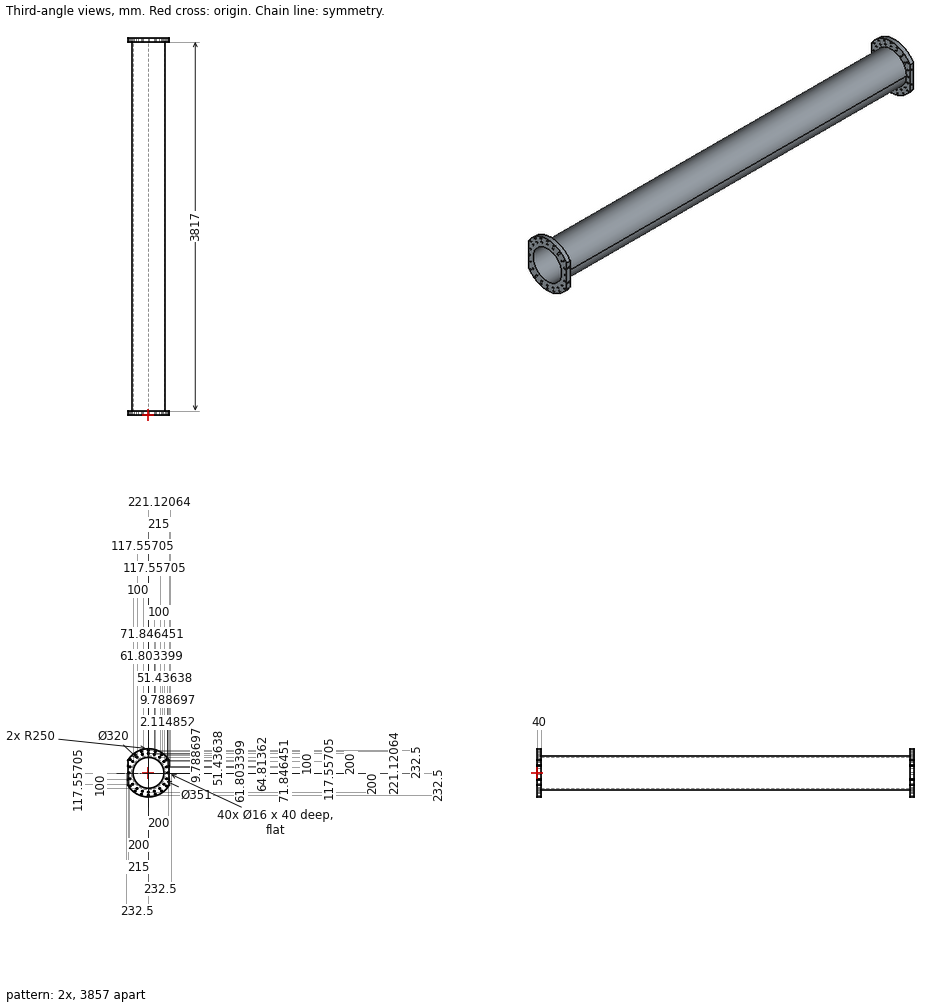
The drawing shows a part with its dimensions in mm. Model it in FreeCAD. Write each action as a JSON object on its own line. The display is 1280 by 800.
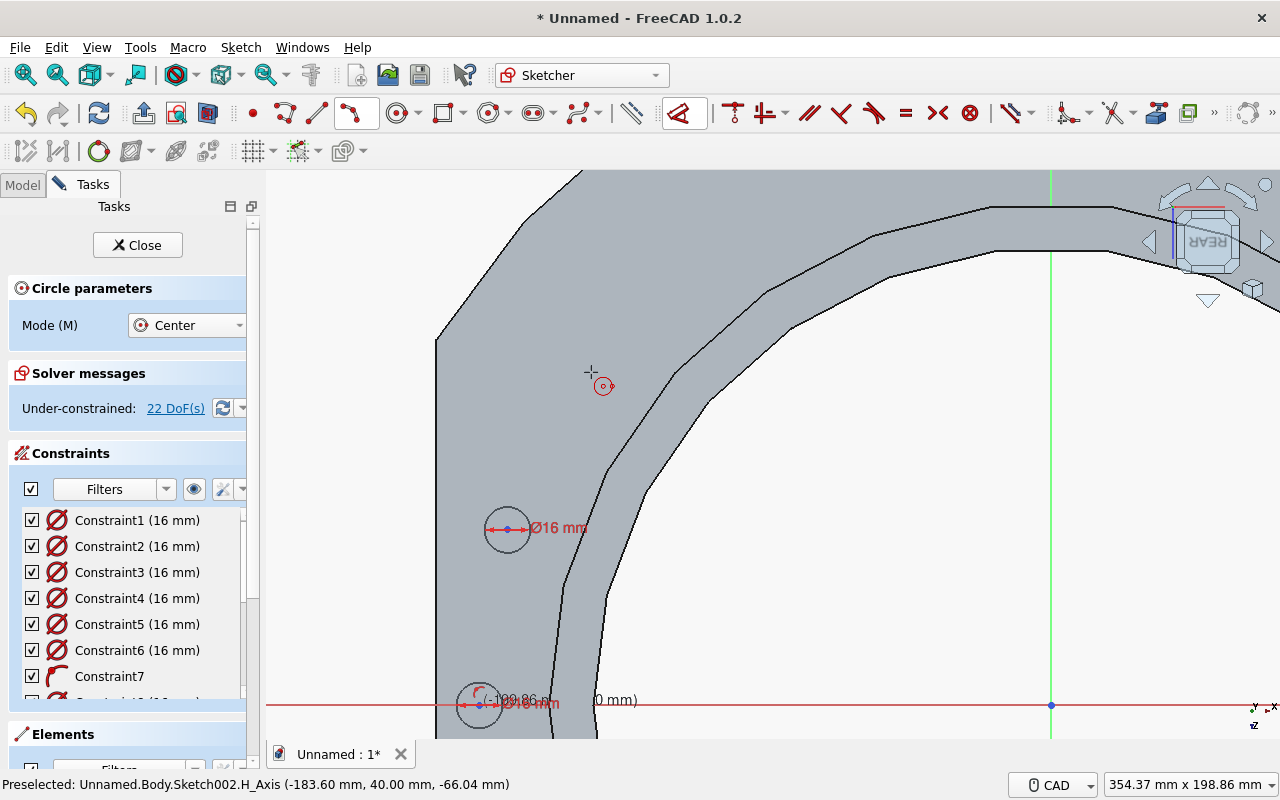
{"action": "left_click", "coordinate": [588, 369]}
{"action": "mouse_move", "coordinate": [605, 353]}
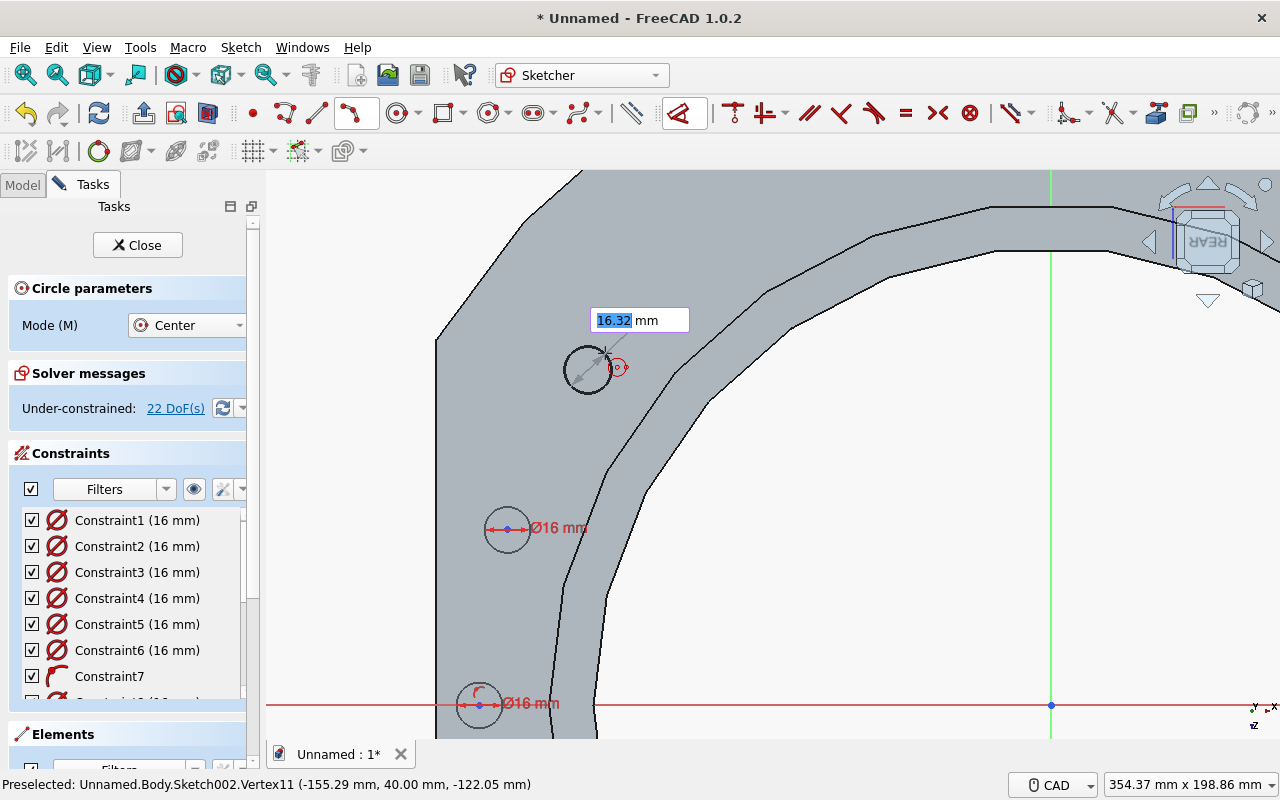
{"action": "type", "text": "16"}
{"action": "key", "text": "Return"}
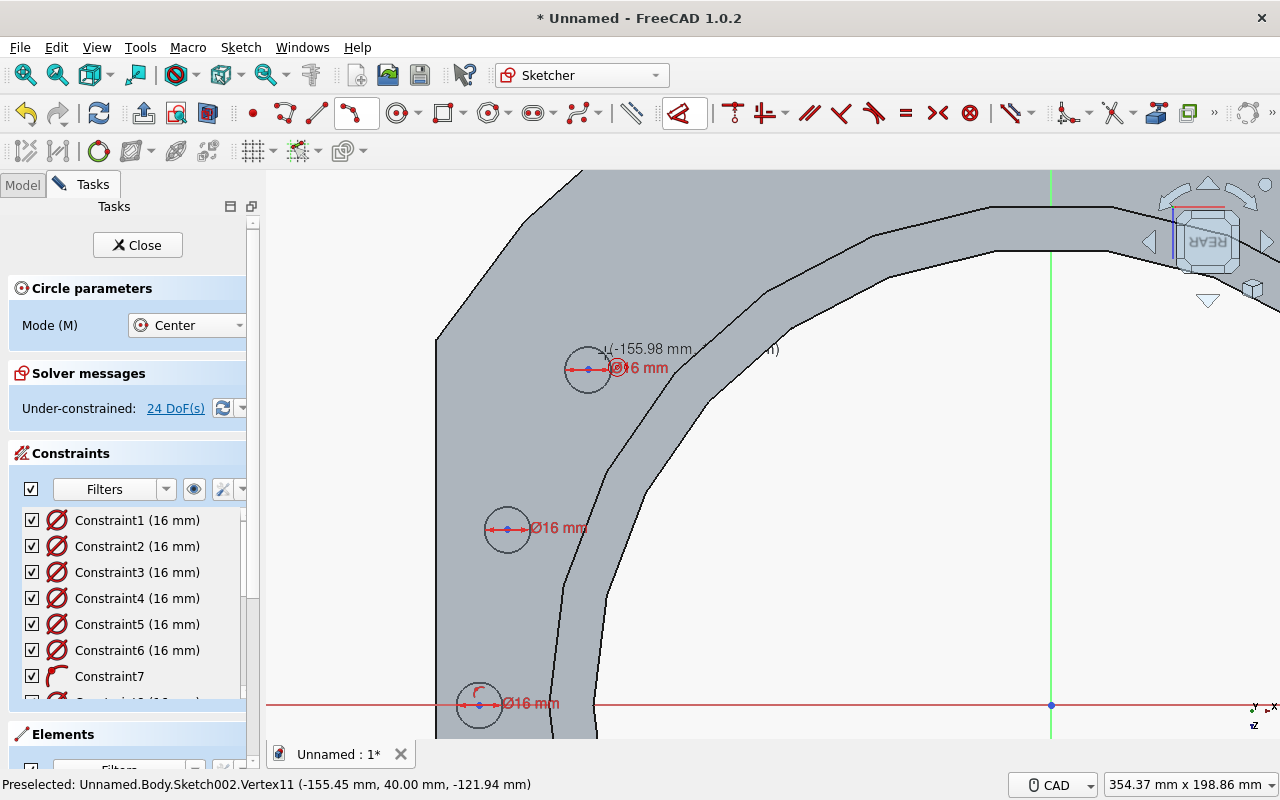
{"action": "left_click", "coordinate": [715, 242]}
{"action": "mouse_move", "coordinate": [731, 226]}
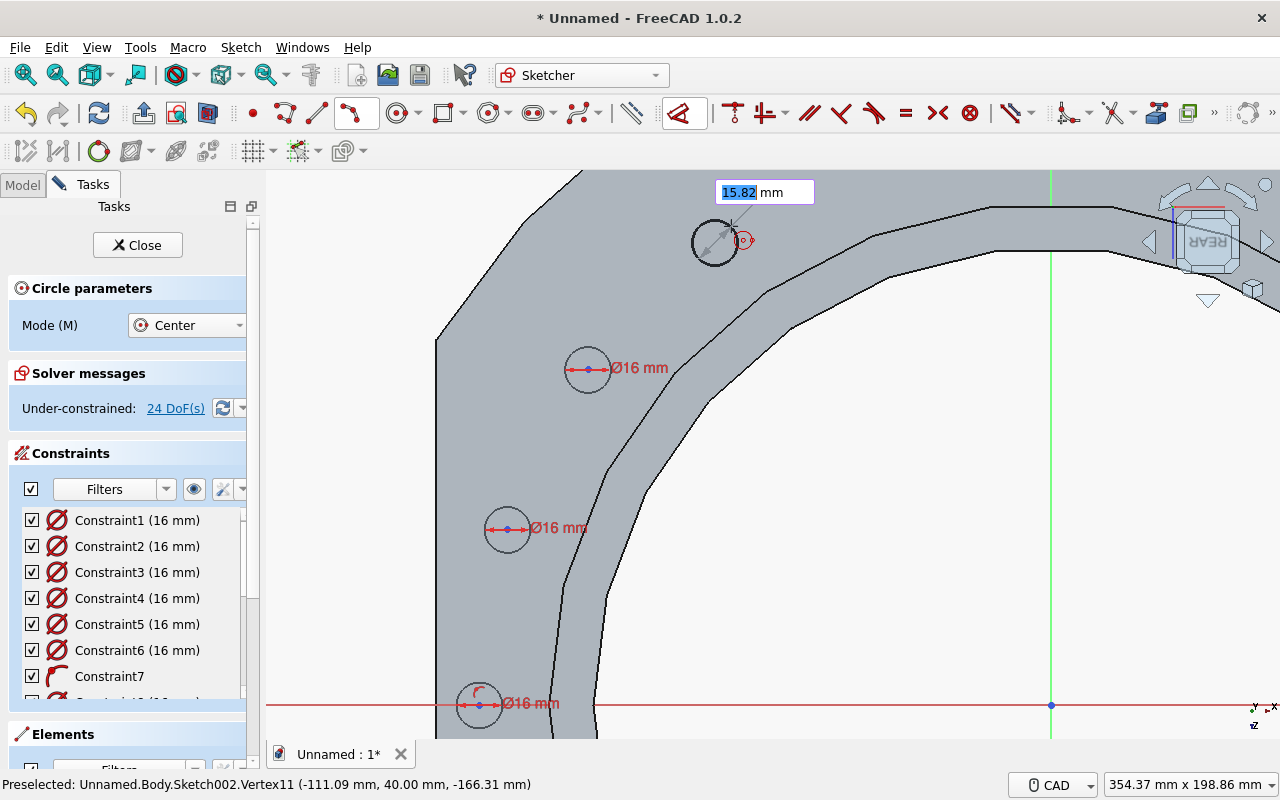
{"action": "type", "text": "16"}
{"action": "key", "text": "Return"}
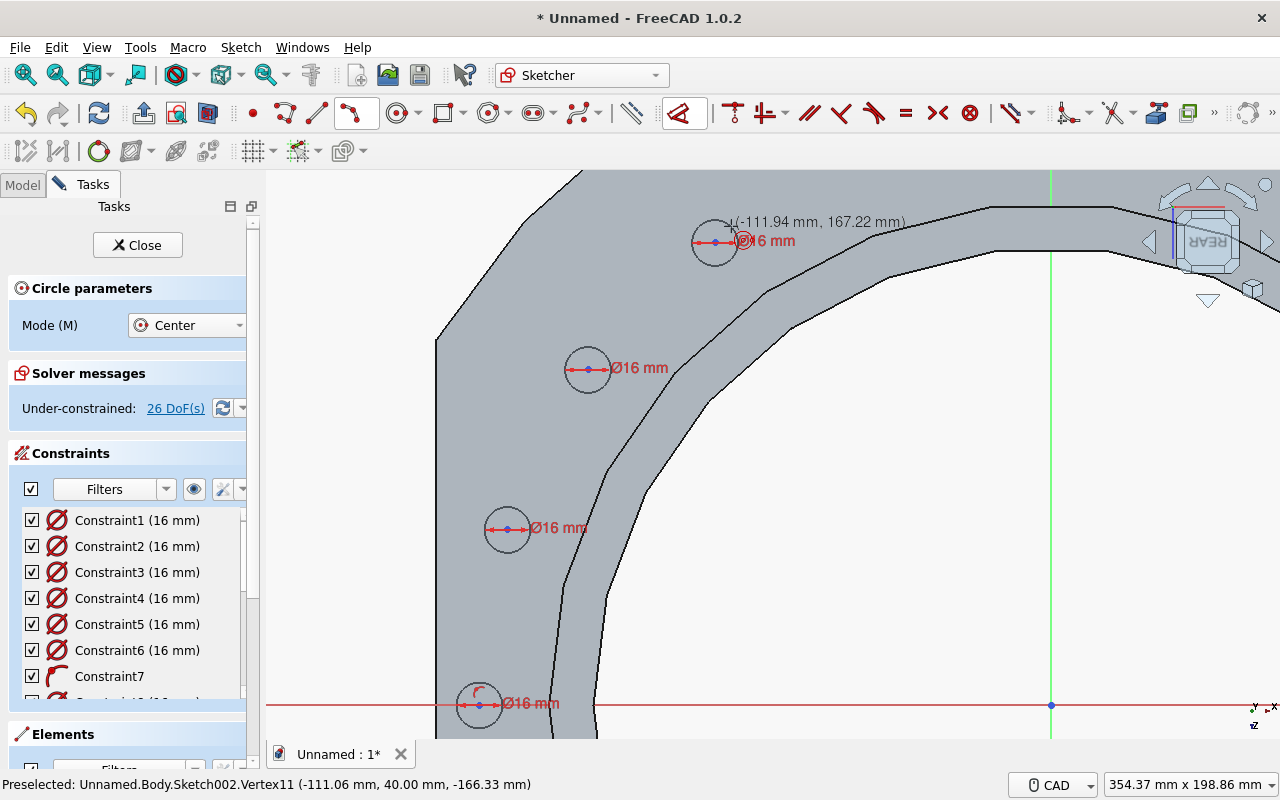
{"action": "scroll", "coordinate": [591, 372], "scroll_direction": "down", "scroll_amount": 7}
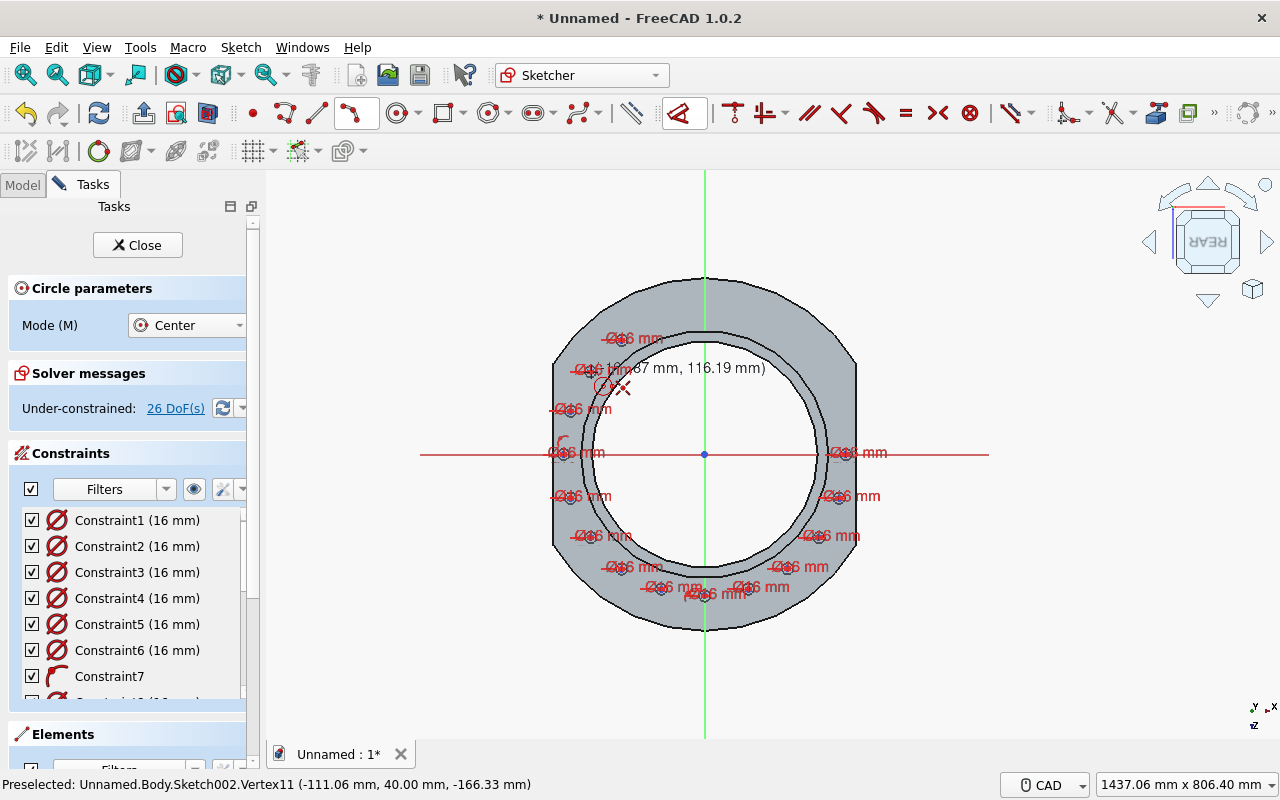
{"action": "scroll", "coordinate": [661, 320], "scroll_direction": "up", "scroll_amount": 7}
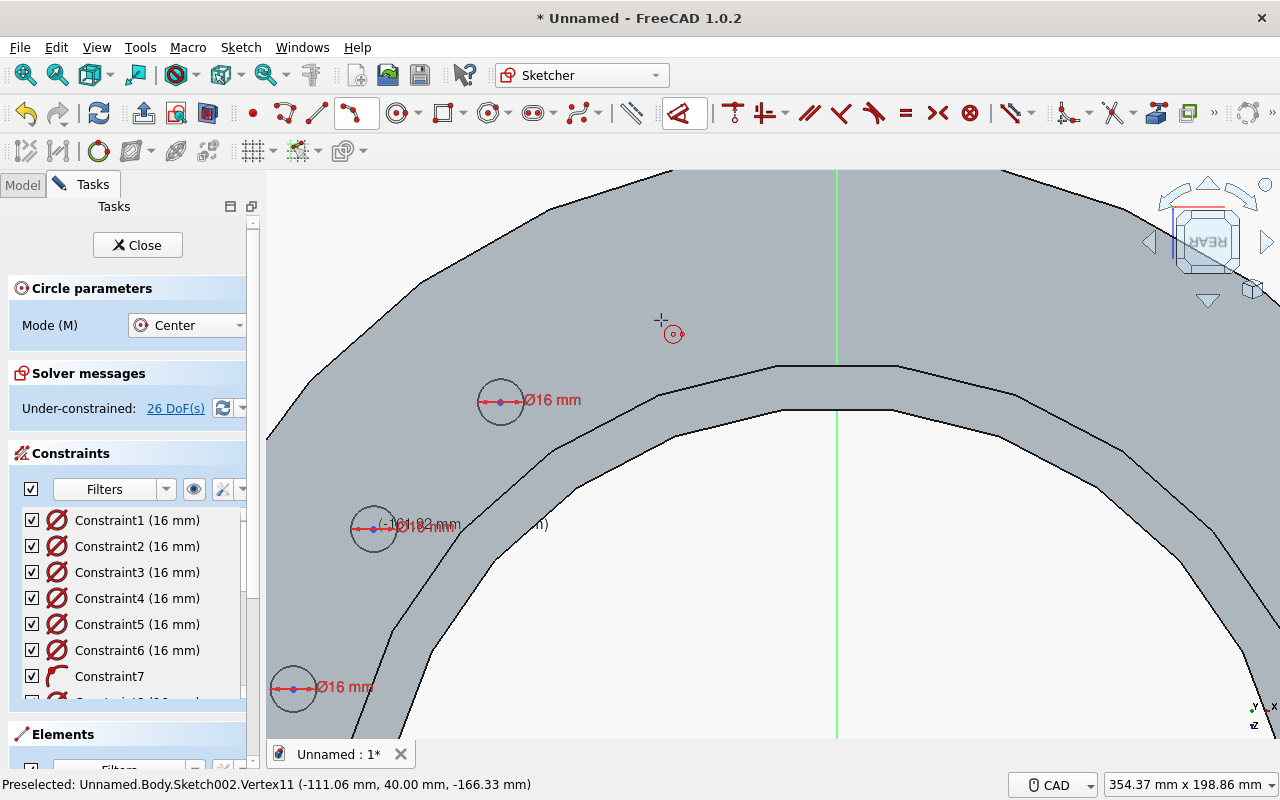
{"action": "left_click", "coordinate": [660, 320]}
{"action": "mouse_move", "coordinate": [677, 304]}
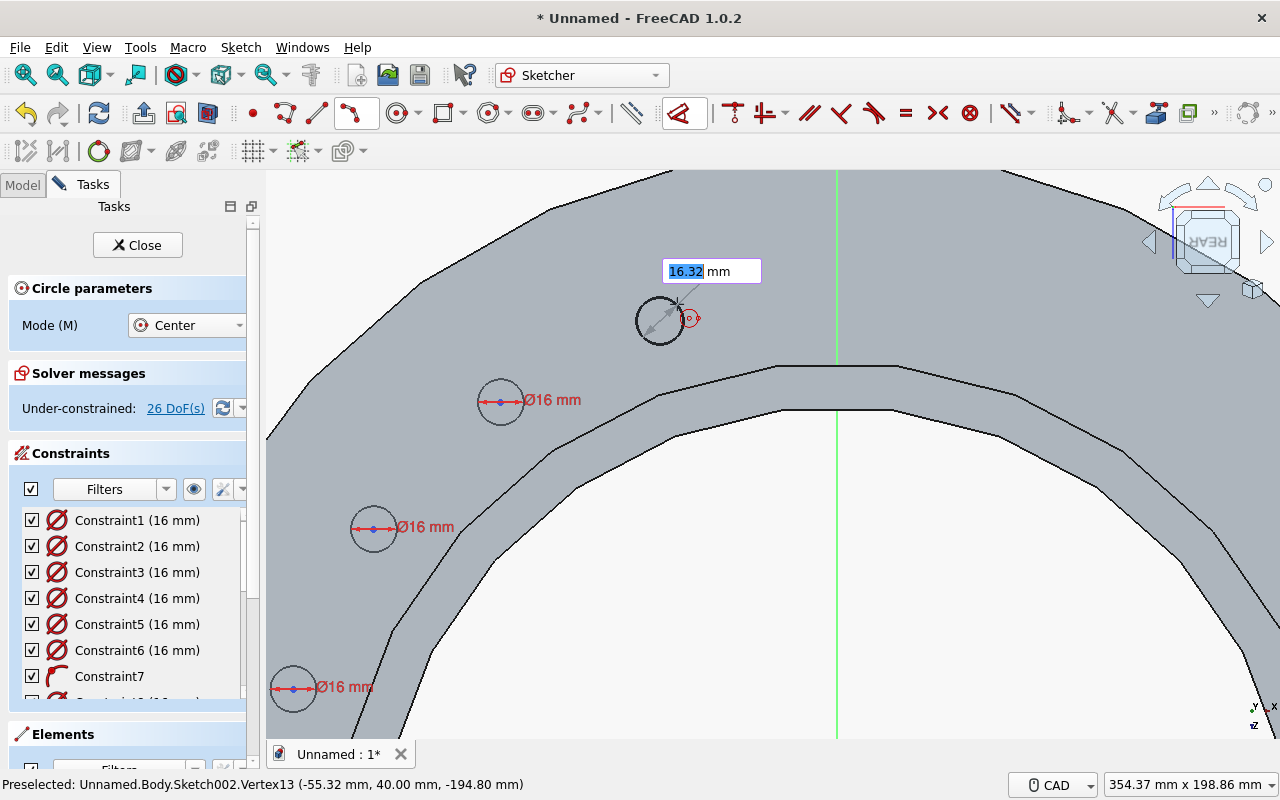
{"action": "type", "text": "16"}
{"action": "key", "text": "Return"}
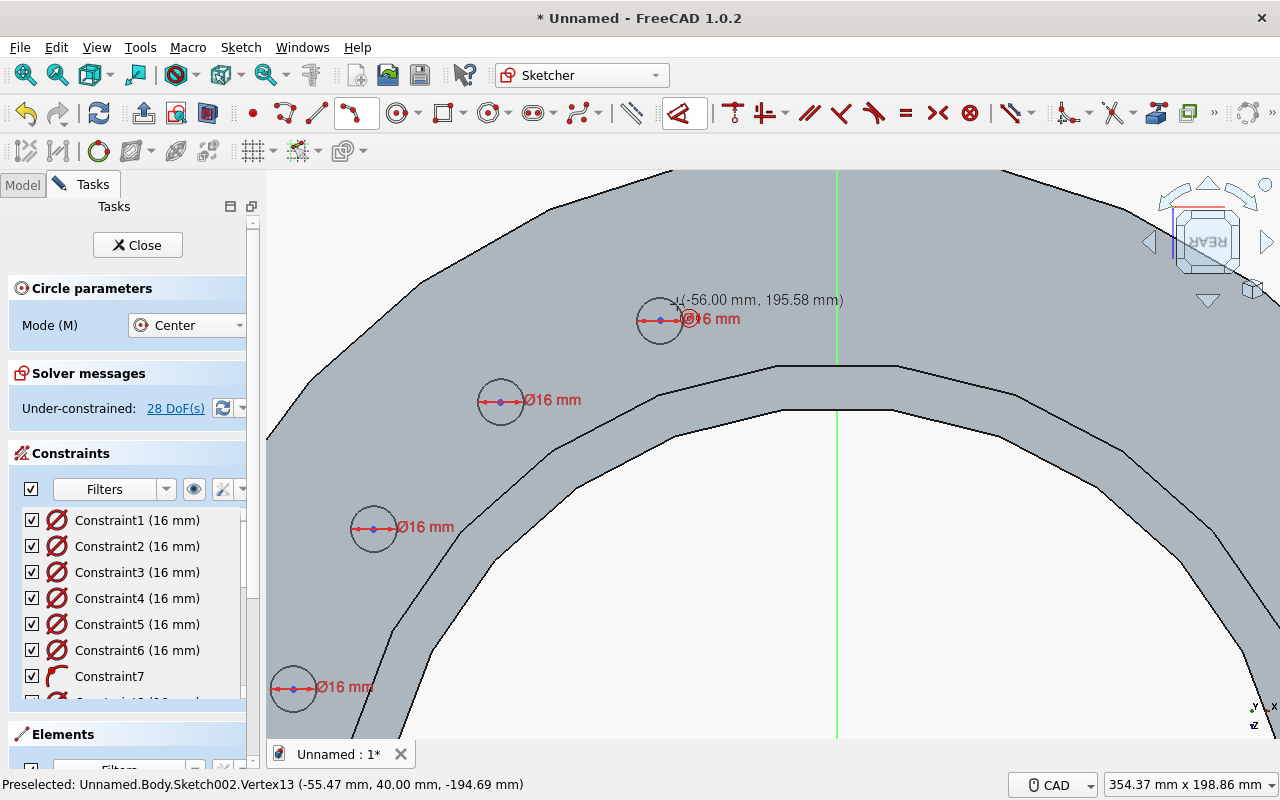
{"action": "left_click", "coordinate": [837, 292]}
{"action": "mouse_move", "coordinate": [853, 276]}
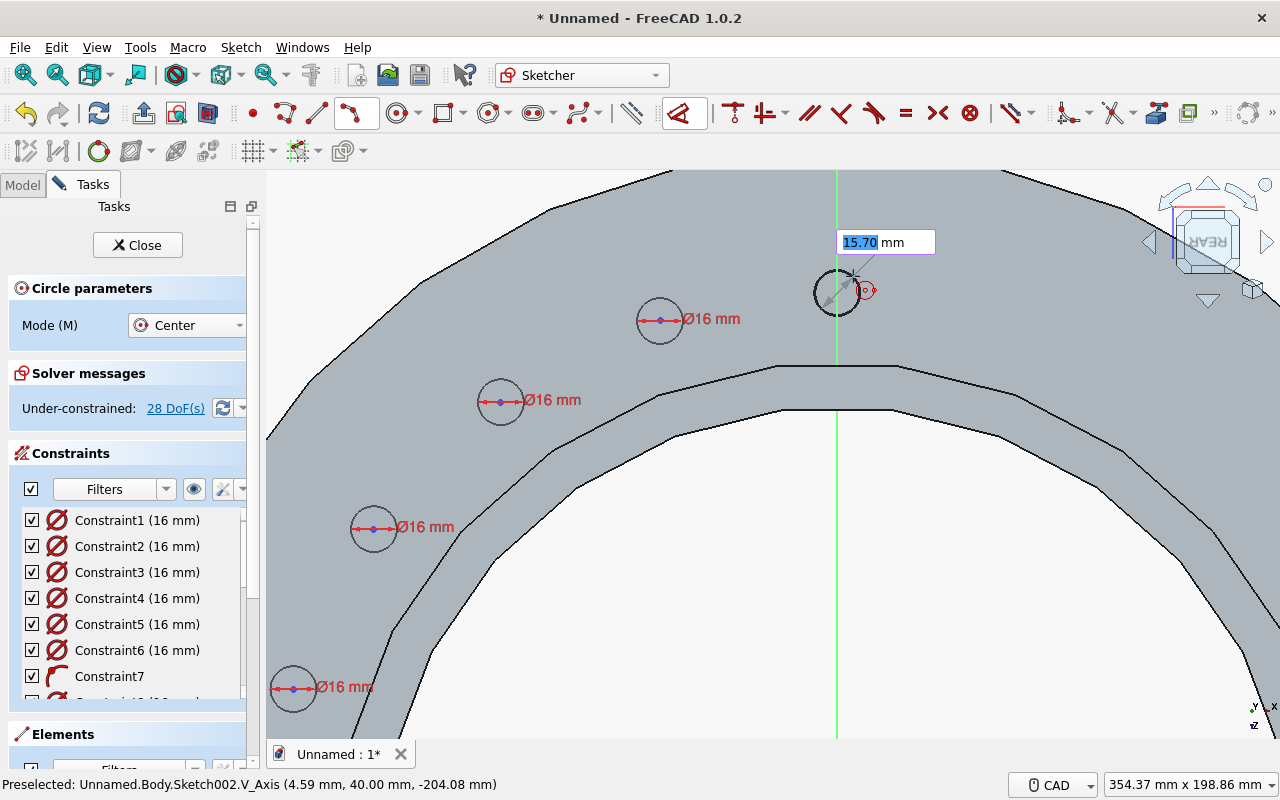
{"action": "type", "text": "16"}
{"action": "key", "text": "Return"}